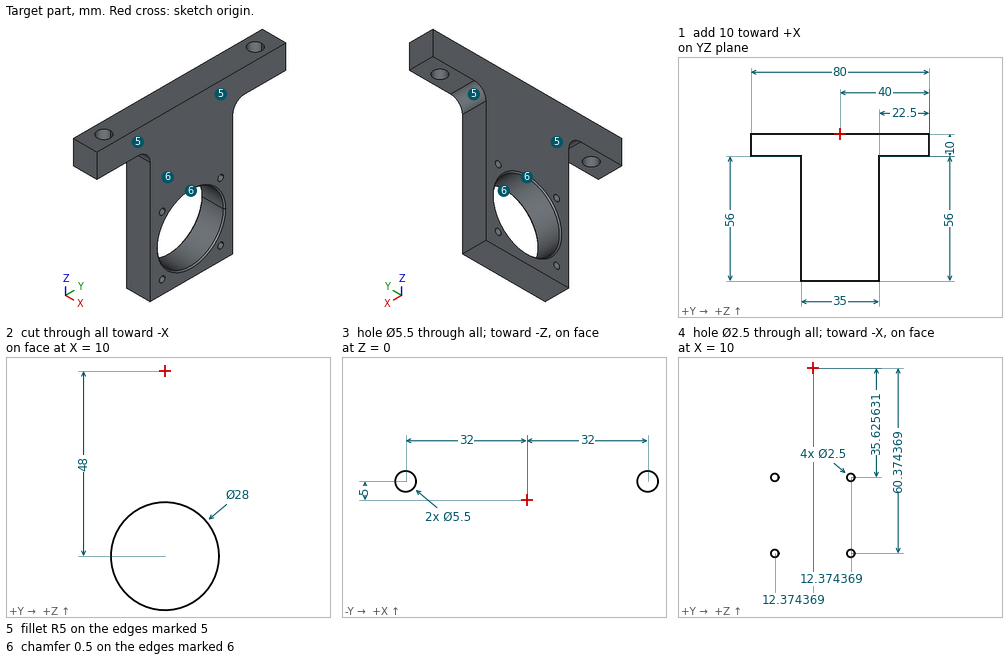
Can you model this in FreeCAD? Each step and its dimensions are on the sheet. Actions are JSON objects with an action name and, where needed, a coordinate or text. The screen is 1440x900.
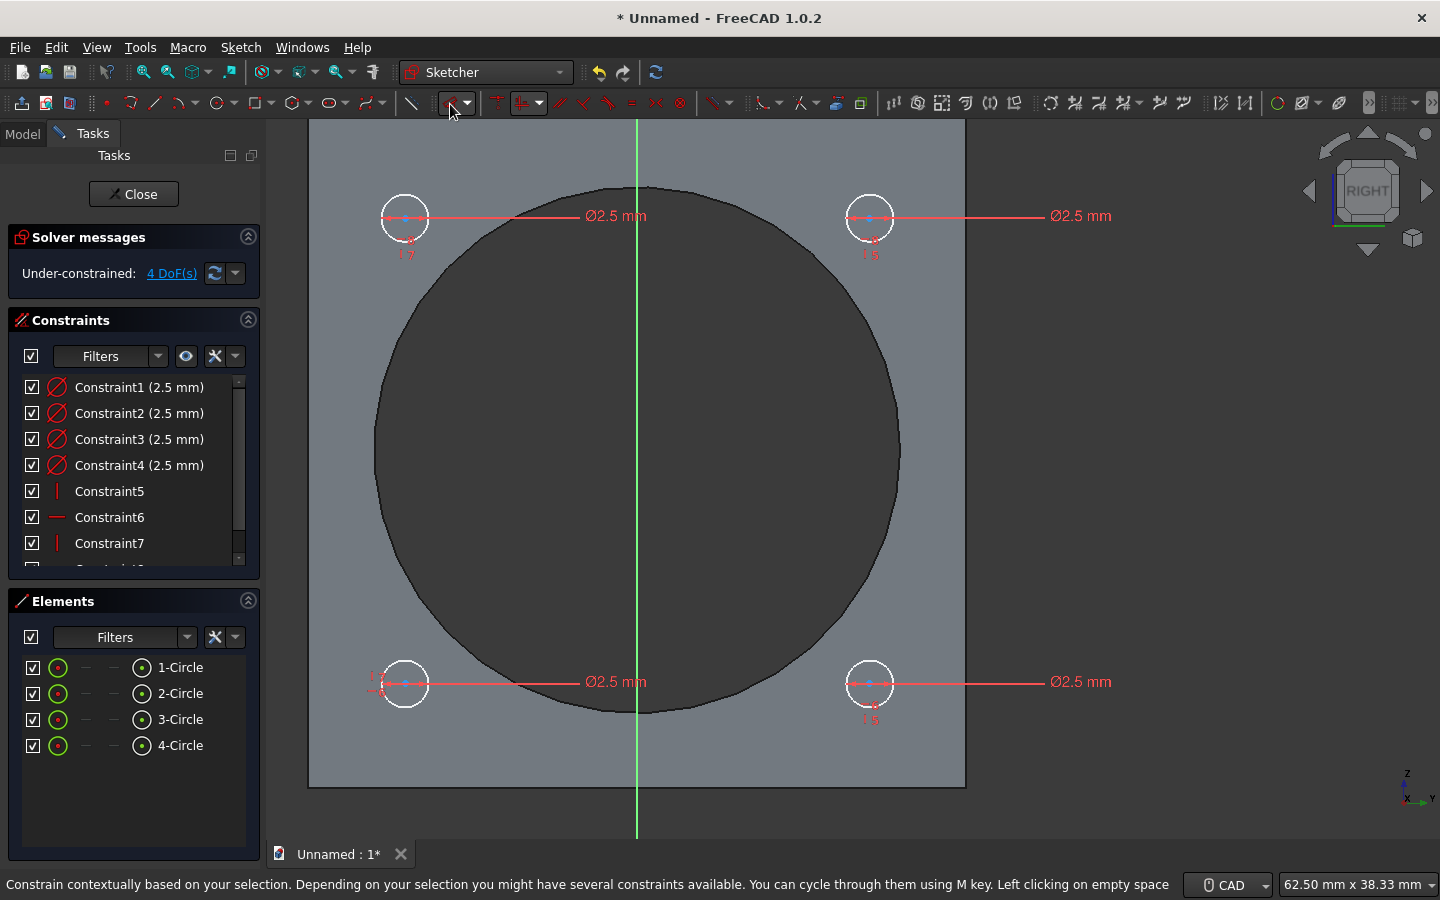
{"action": "left_click", "coordinate": [870, 218]}
{"action": "left_click", "coordinate": [754, 252]}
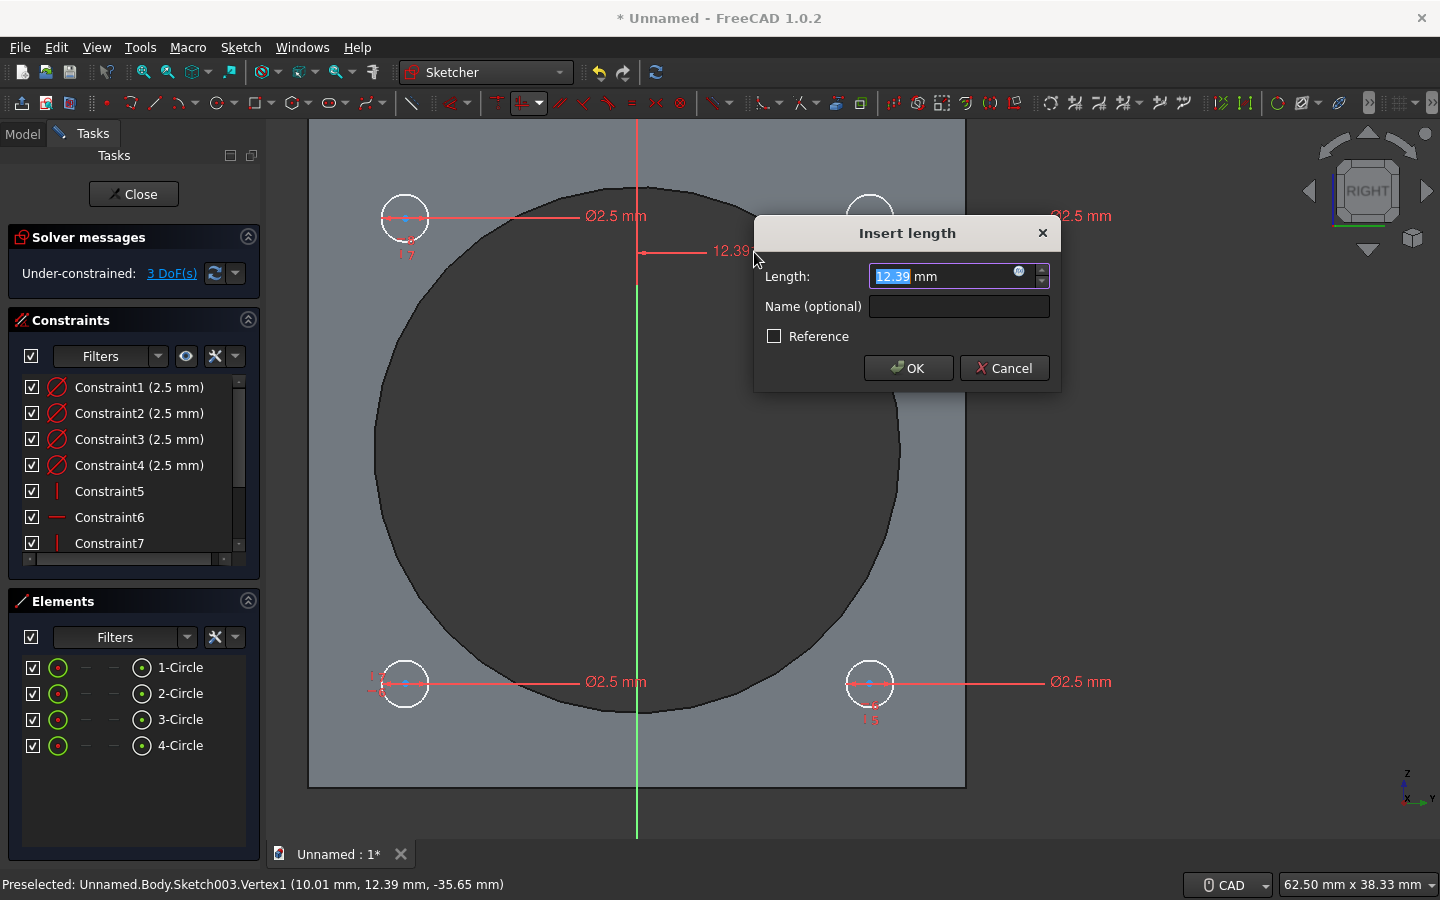
{"action": "type", "text": "12.374369"}
{"action": "key", "text": "Return"}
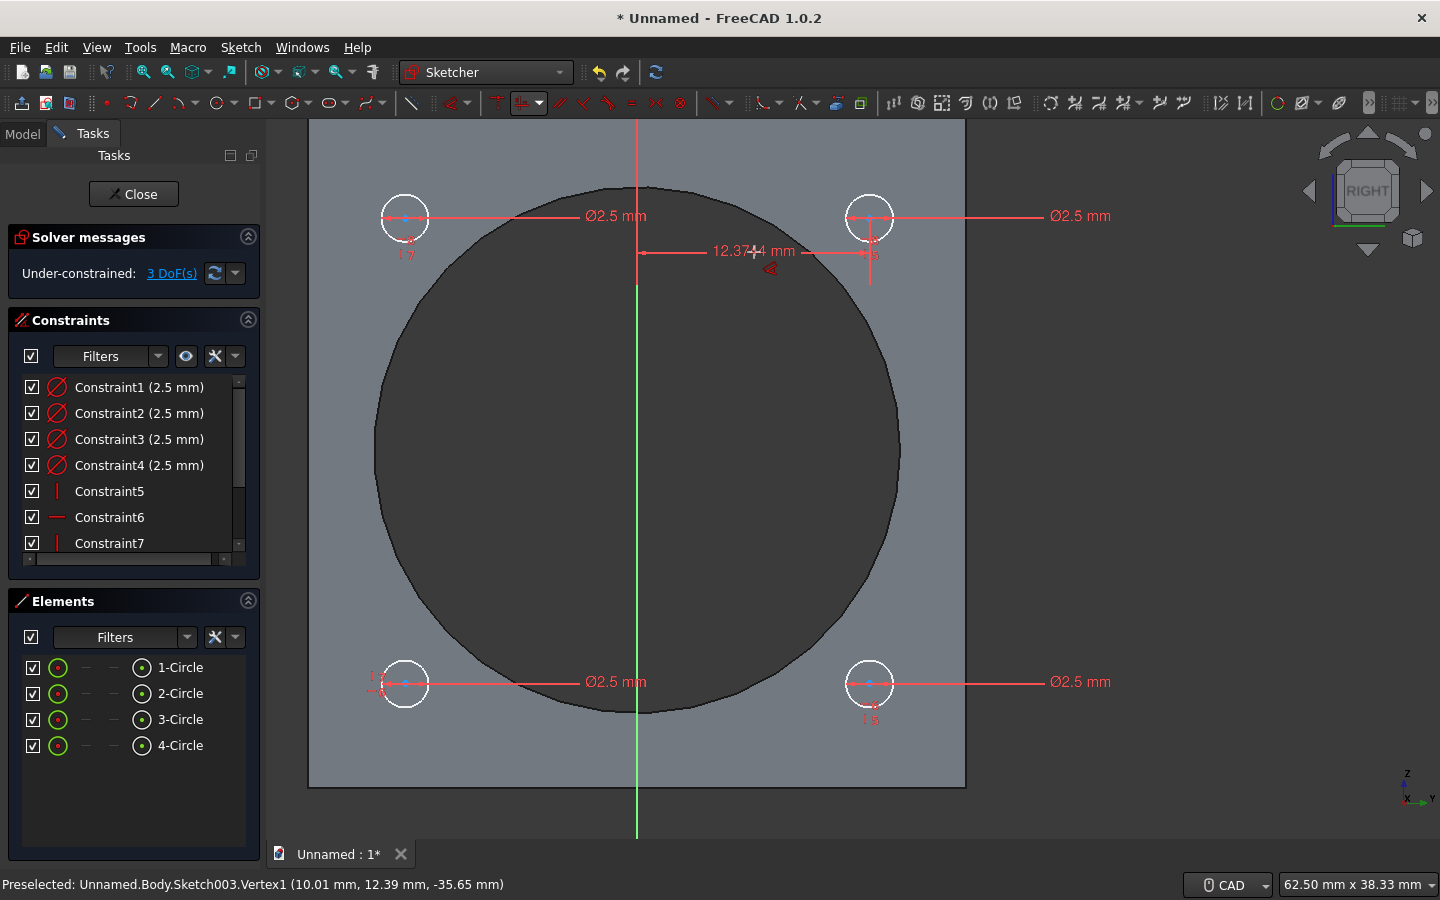
{"action": "left_click", "coordinate": [870, 218]}
{"action": "left_click", "coordinate": [904, 183]}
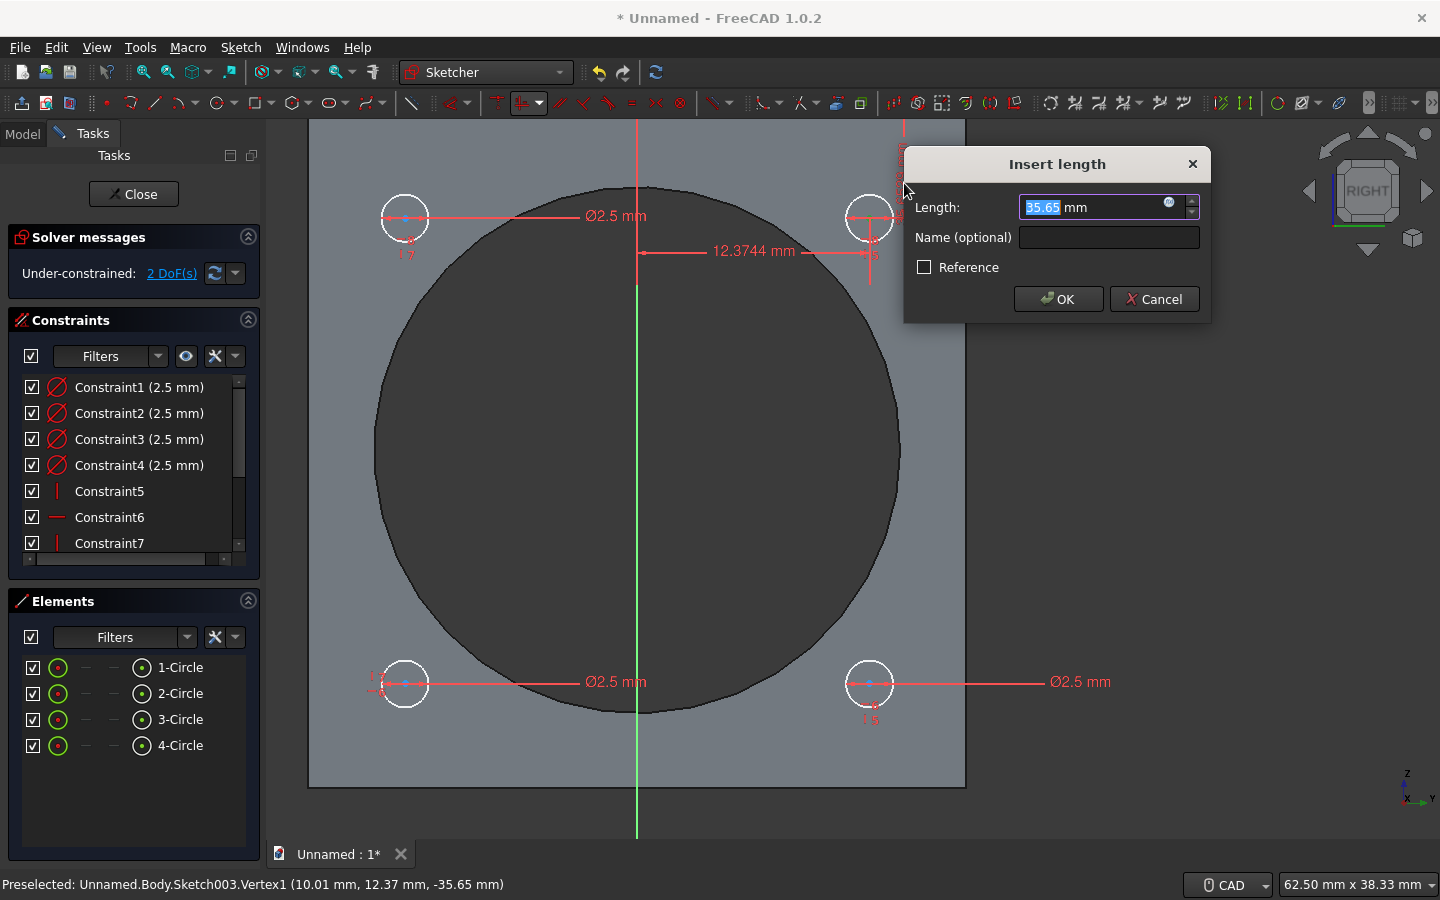
{"action": "type", "text": "35.625631"}
{"action": "key", "text": "Return"}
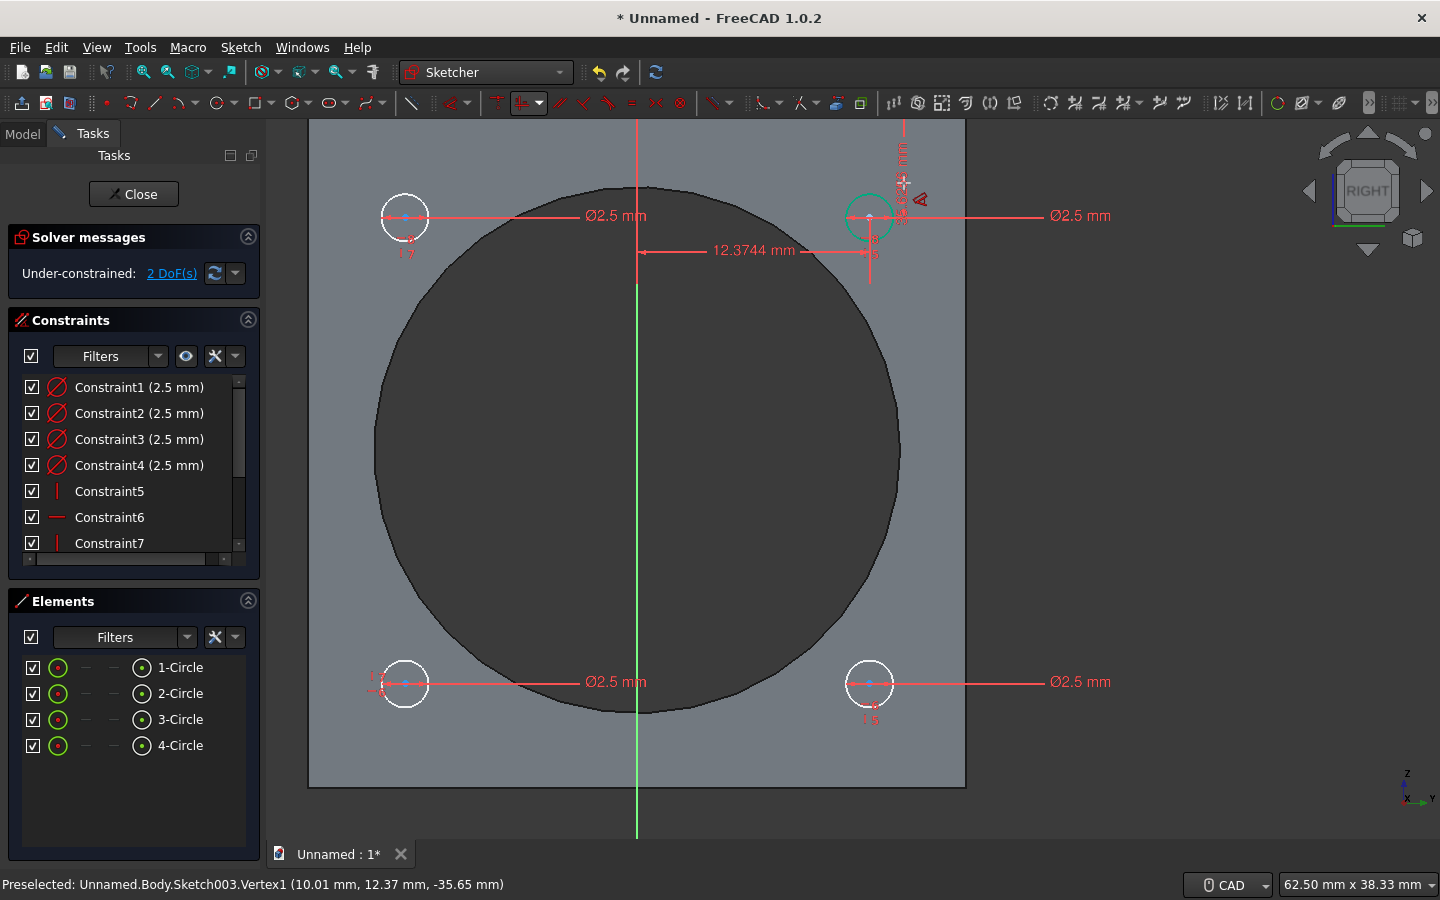
{"action": "left_click", "coordinate": [870, 684]}
{"action": "left_click", "coordinate": [904, 416]}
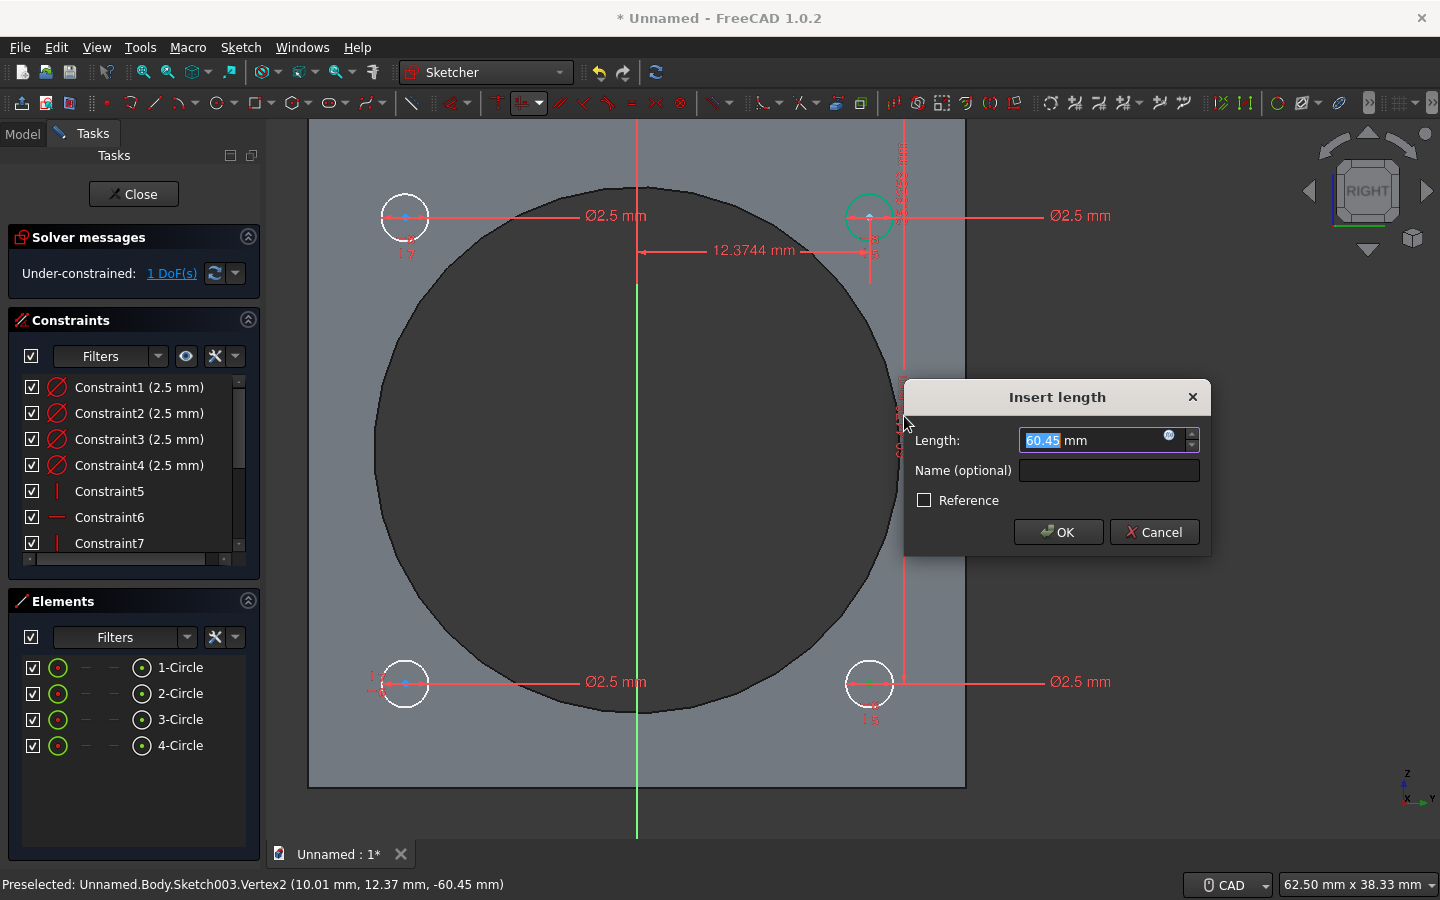
{"action": "type", "text": "60.374369"}
{"action": "key", "text": "Return"}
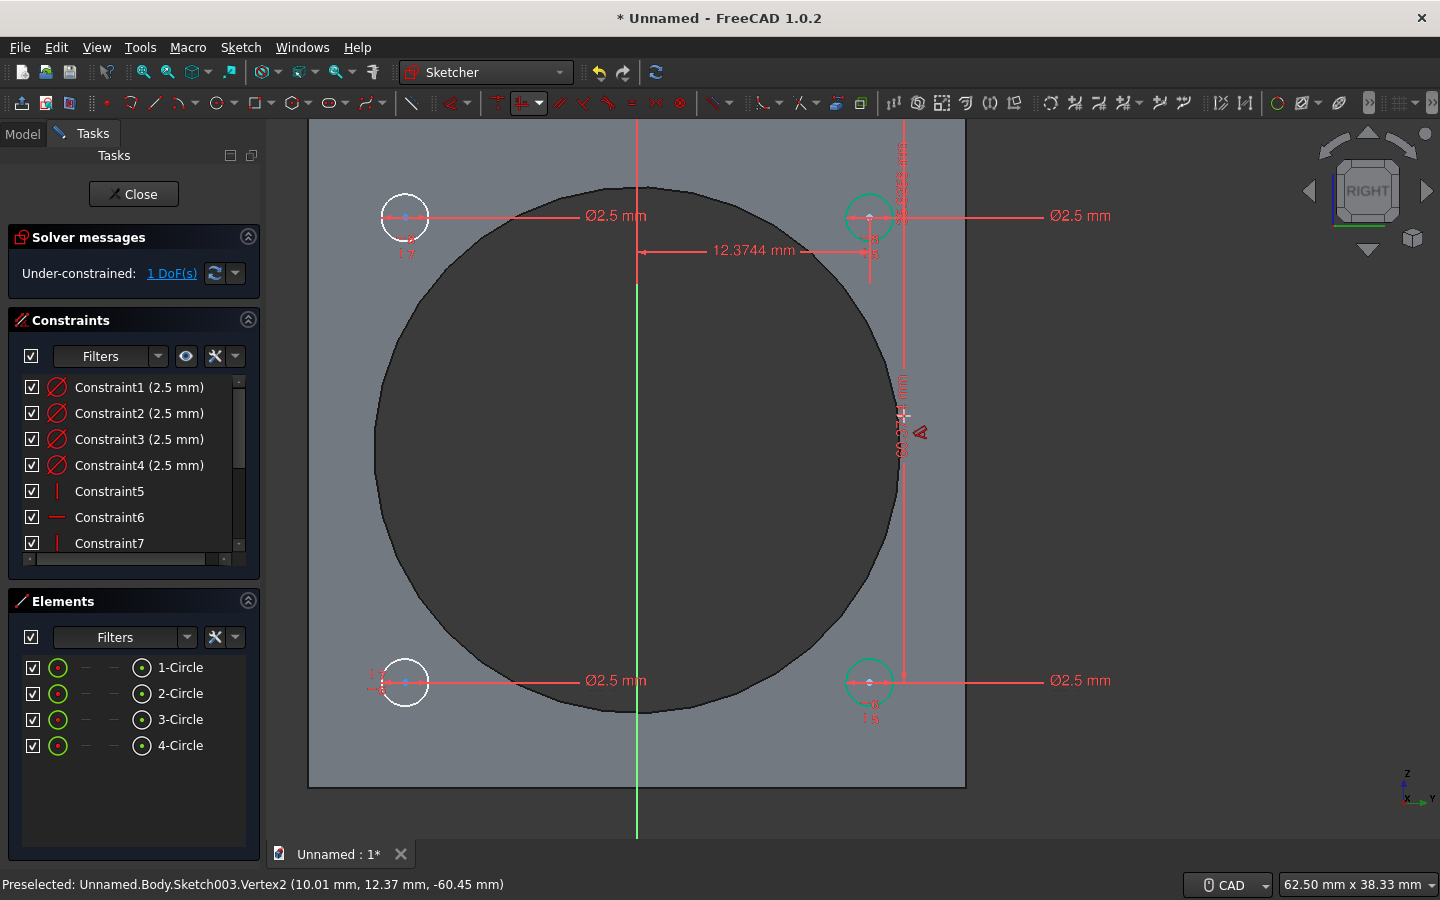
{"action": "left_click", "coordinate": [405, 683]}
{"action": "left_click", "coordinate": [521, 717]}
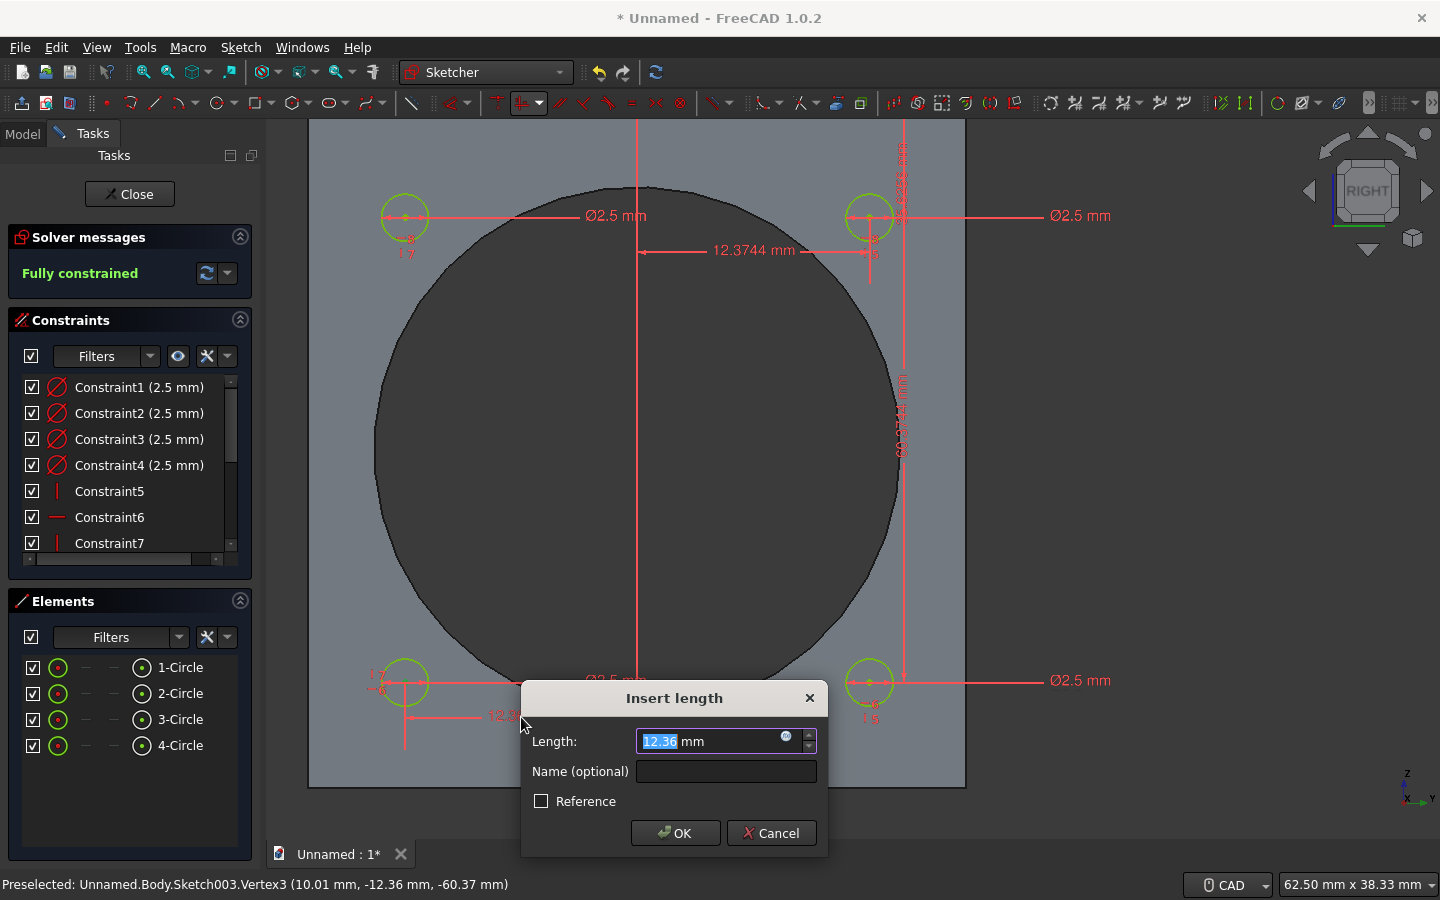
{"action": "type", "text": "12.374369"}
{"action": "key", "text": "Return"}
{"action": "key", "text": "Escape"}